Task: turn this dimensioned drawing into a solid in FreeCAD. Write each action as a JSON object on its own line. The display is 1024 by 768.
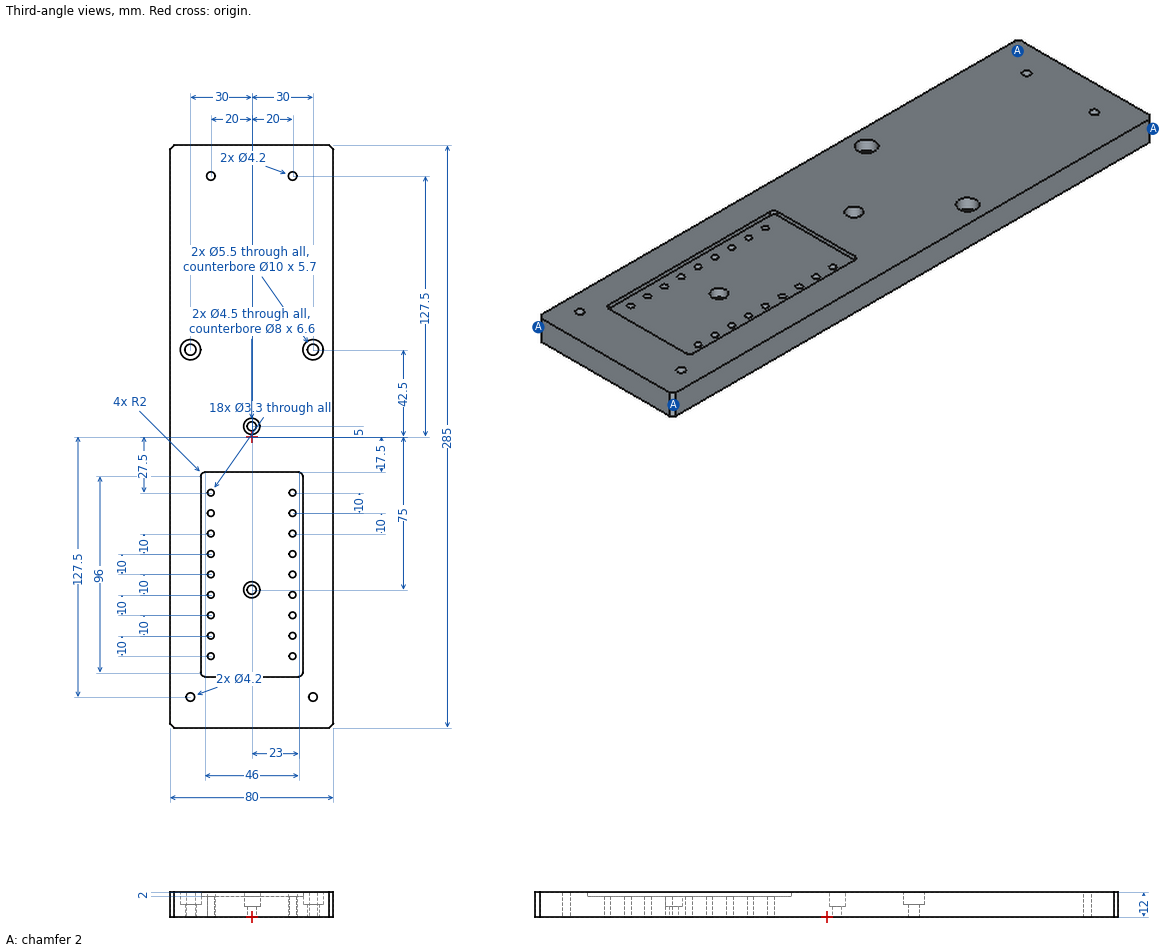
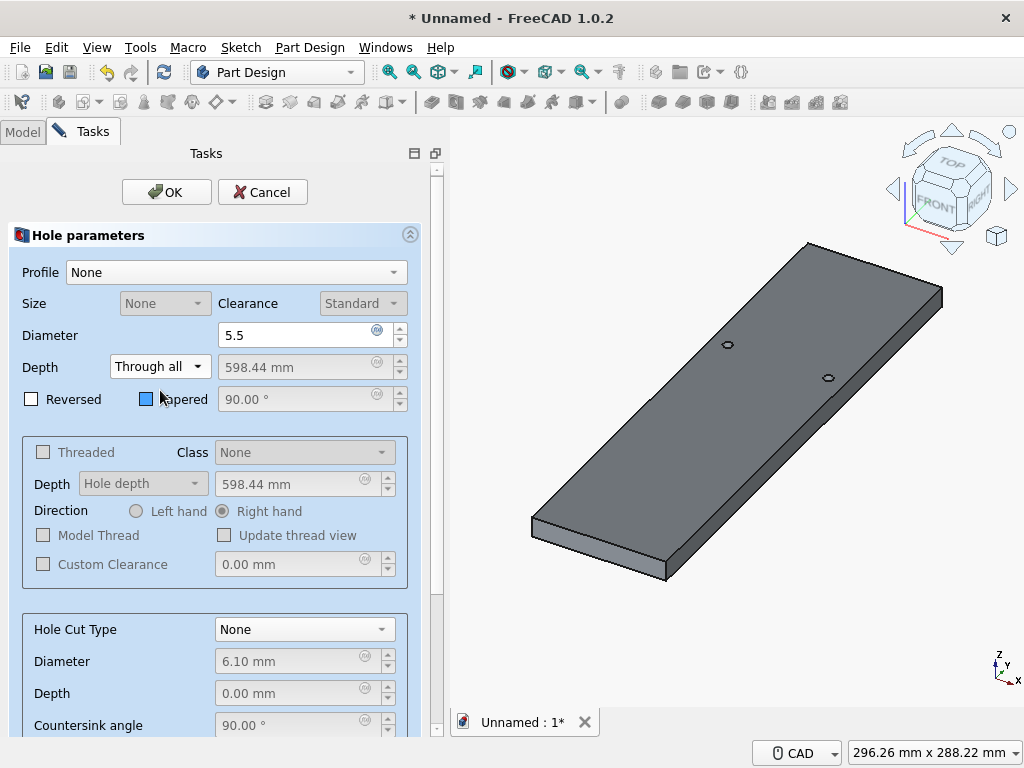
{"action": "left_click", "coordinate": [306, 630]}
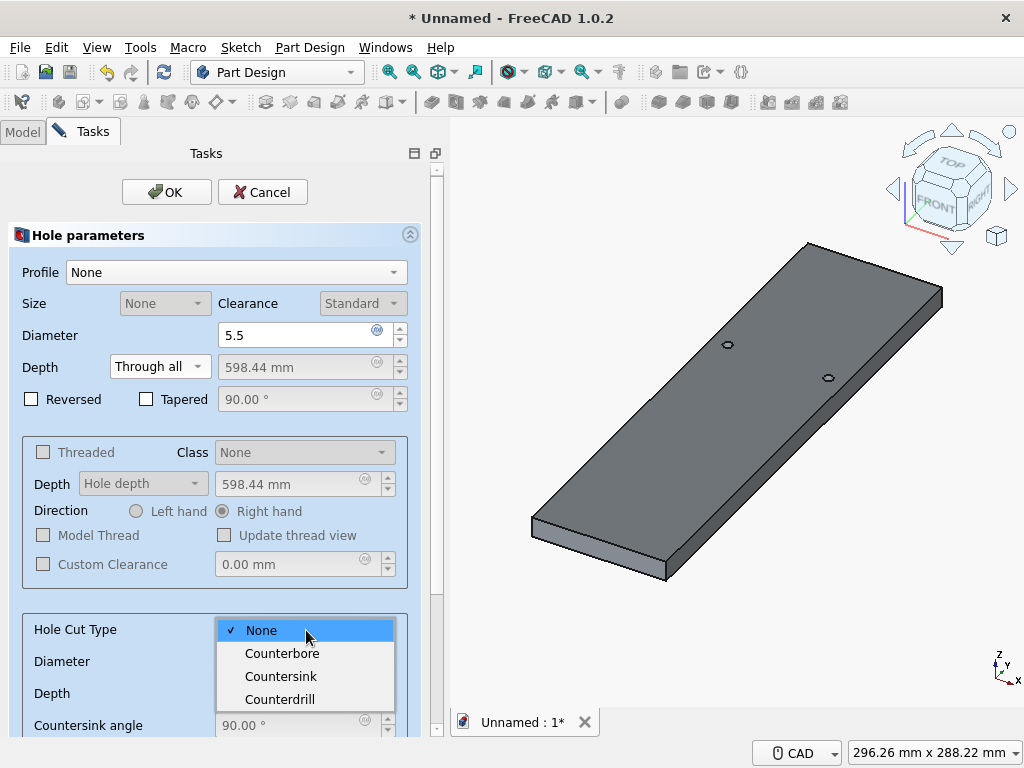
{"action": "left_click", "coordinate": [304, 654]}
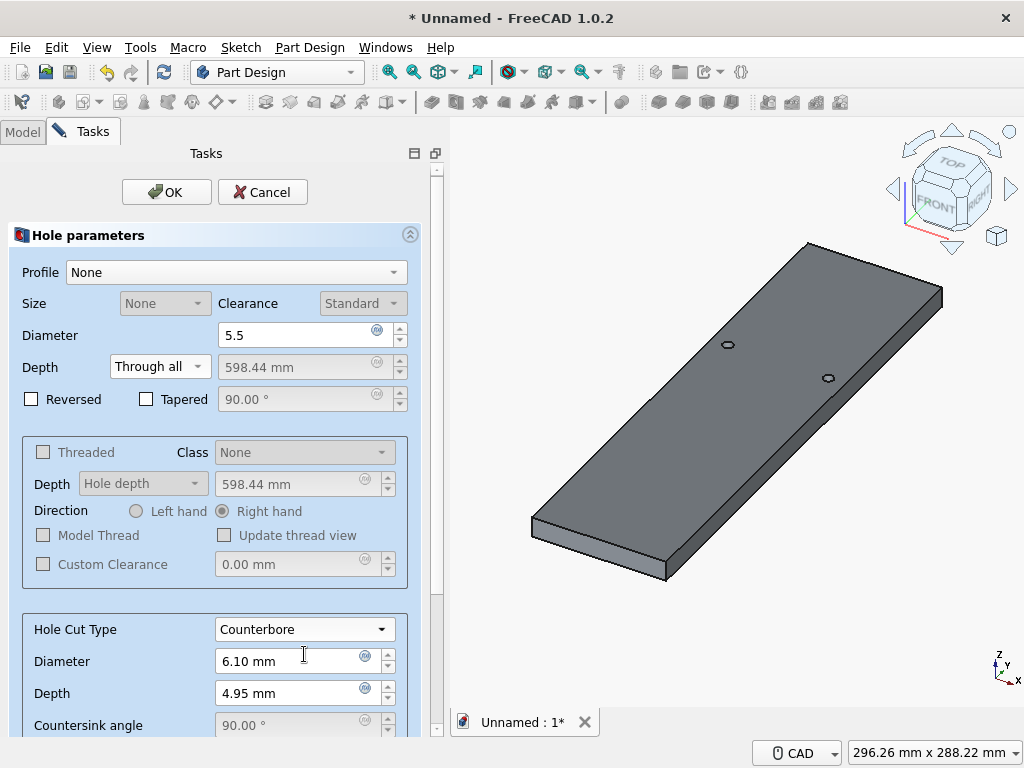
{"action": "triple_click", "coordinate": [298, 661]}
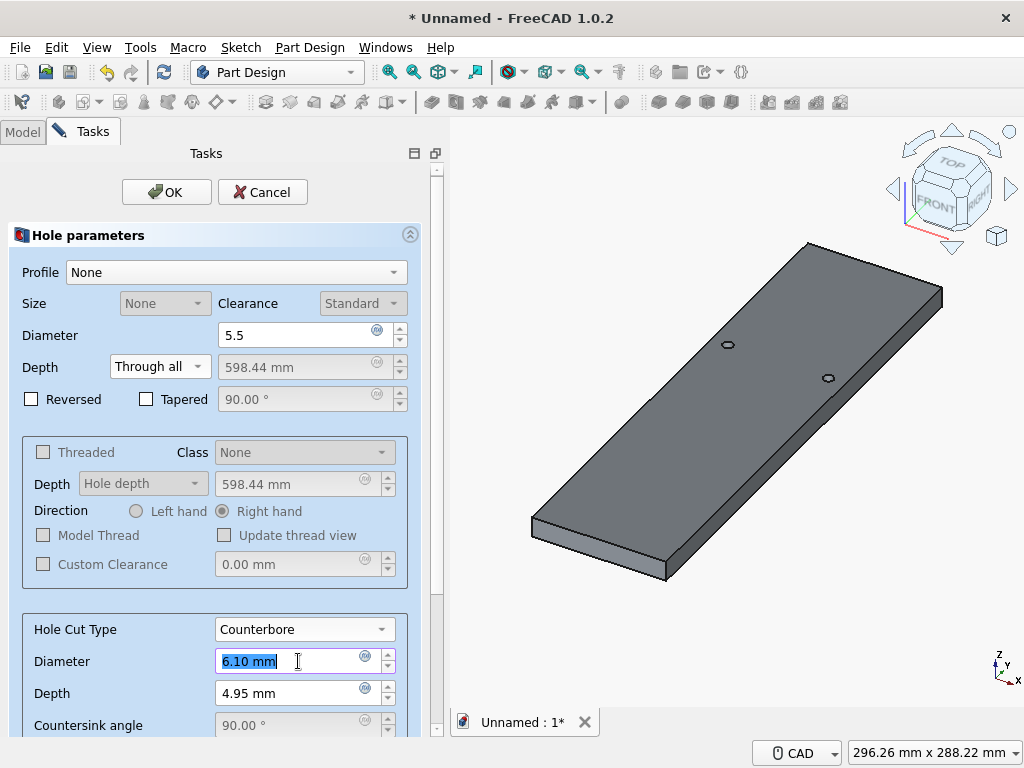
{"action": "type", "text": "10"}
{"action": "key", "text": "Tab"}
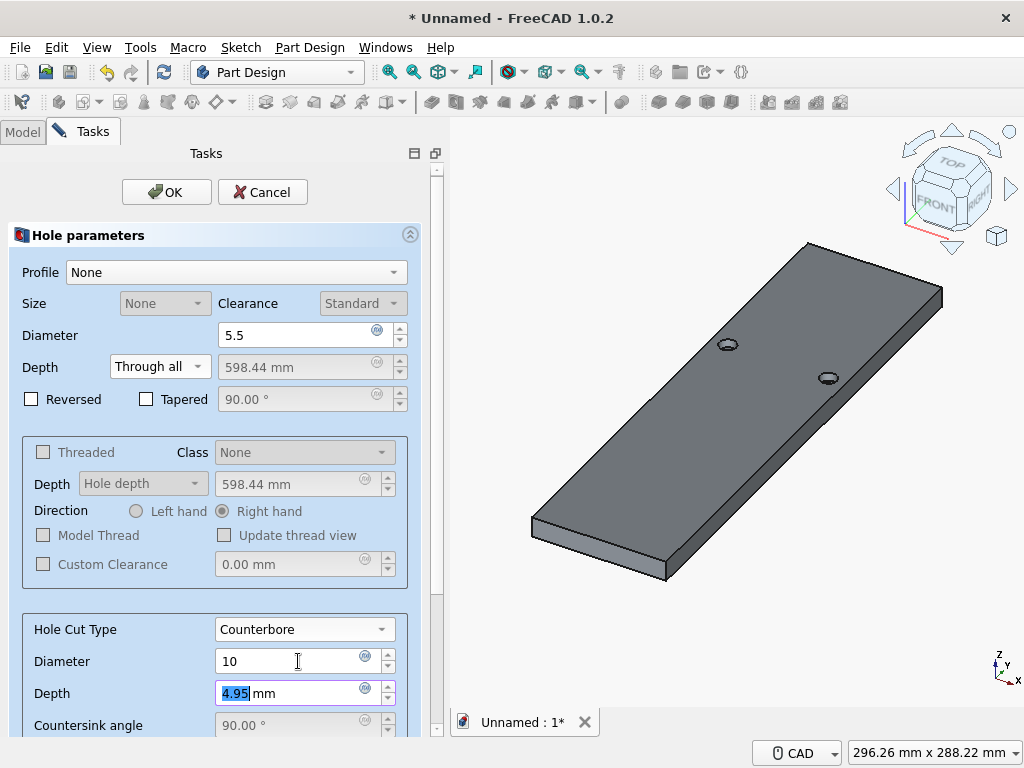
{"action": "type", "text": "5.7"}
{"action": "key", "text": "Tab"}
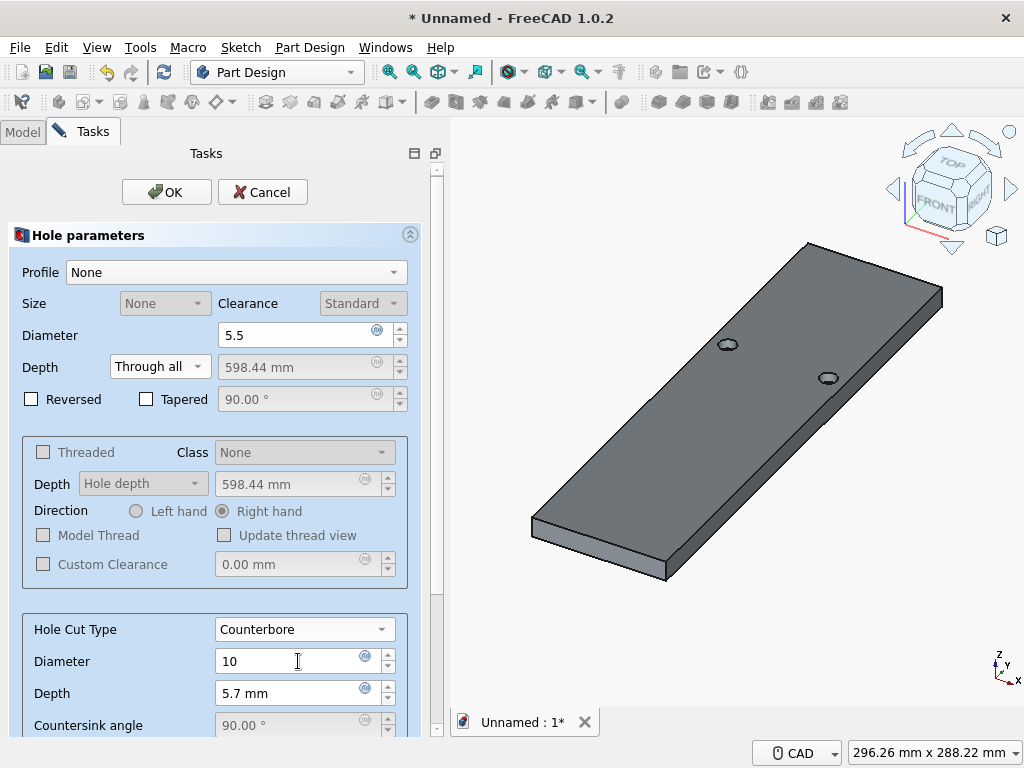
{"action": "left_click", "coordinate": [167, 192]}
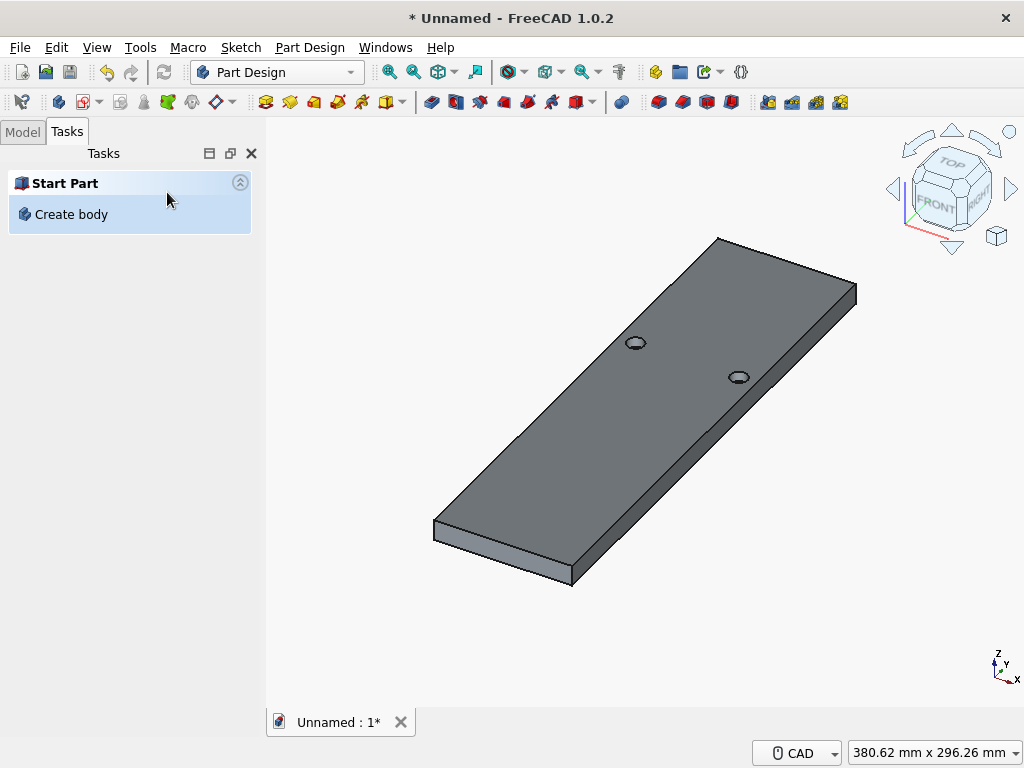
{"action": "key", "text": "5"}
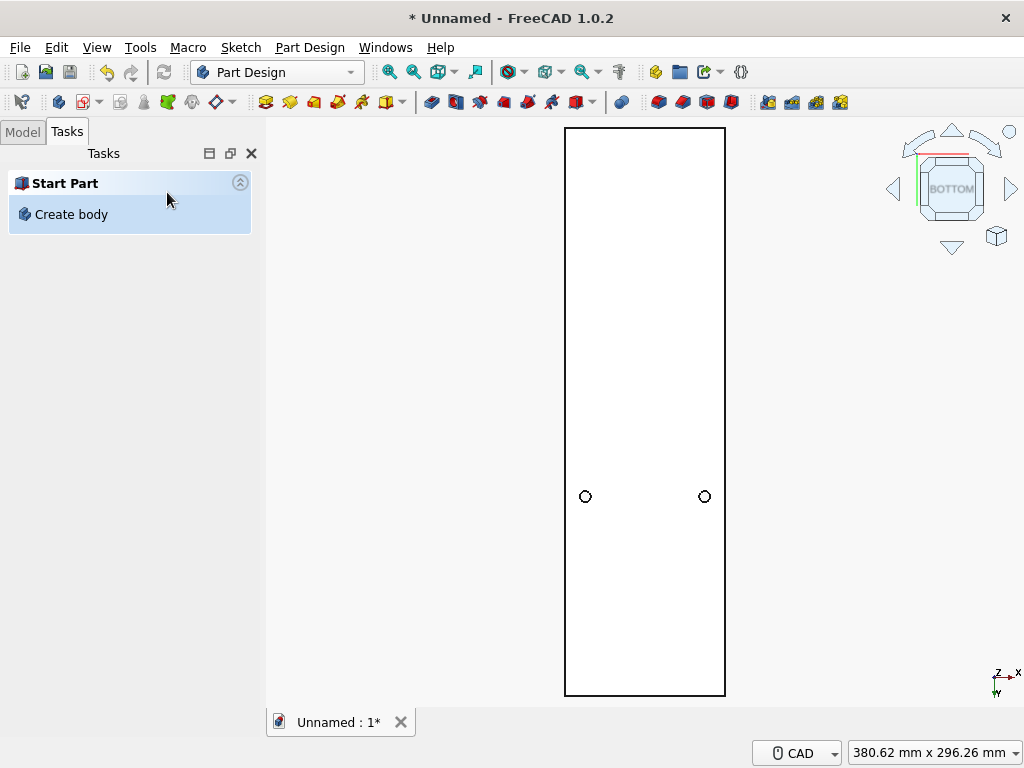
{"action": "left_click", "coordinate": [645, 573]}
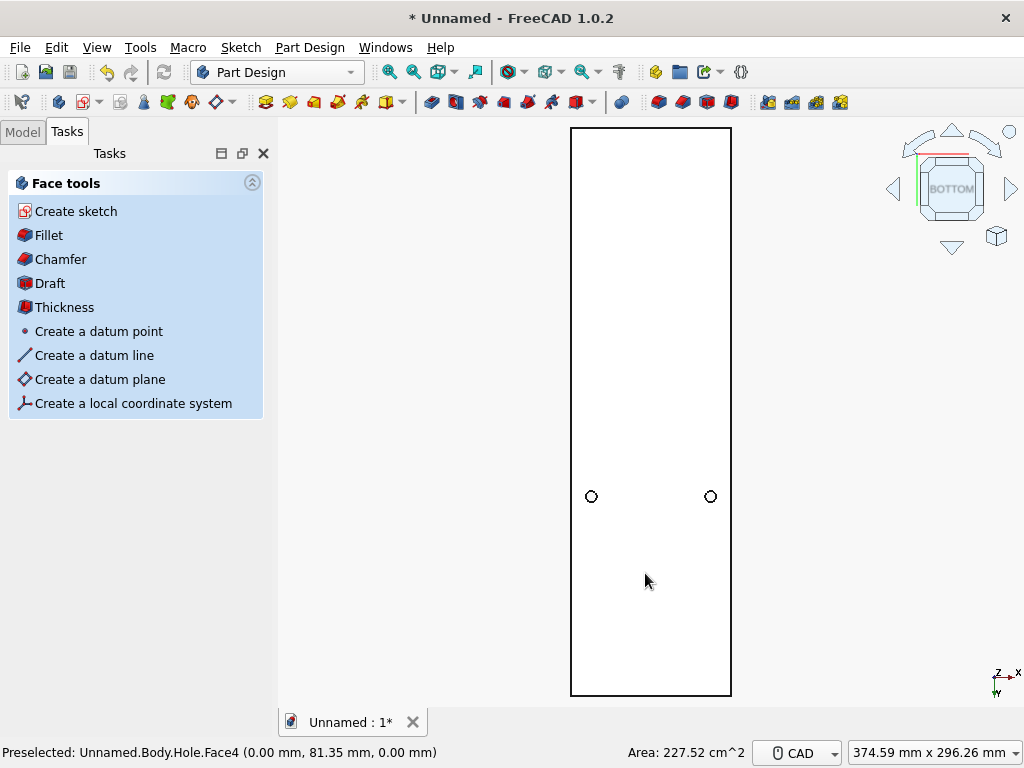
{"action": "left_click", "coordinate": [84, 102]}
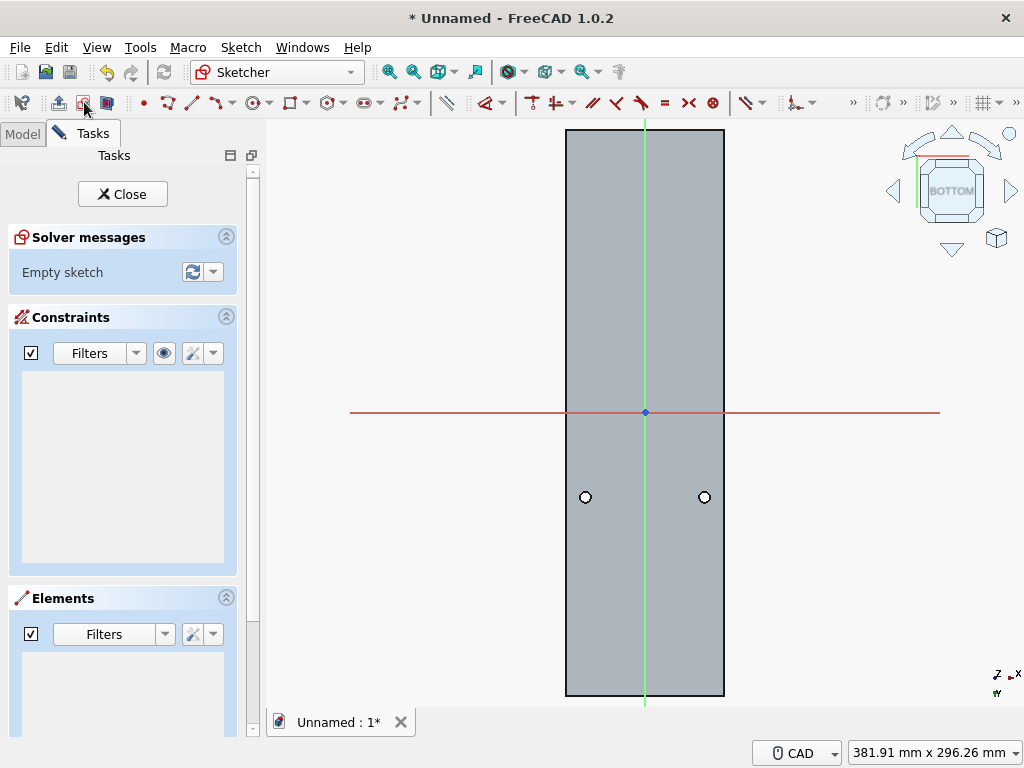
{"action": "scroll", "coordinate": [662, 679], "scroll_direction": "up", "scroll_amount": 8}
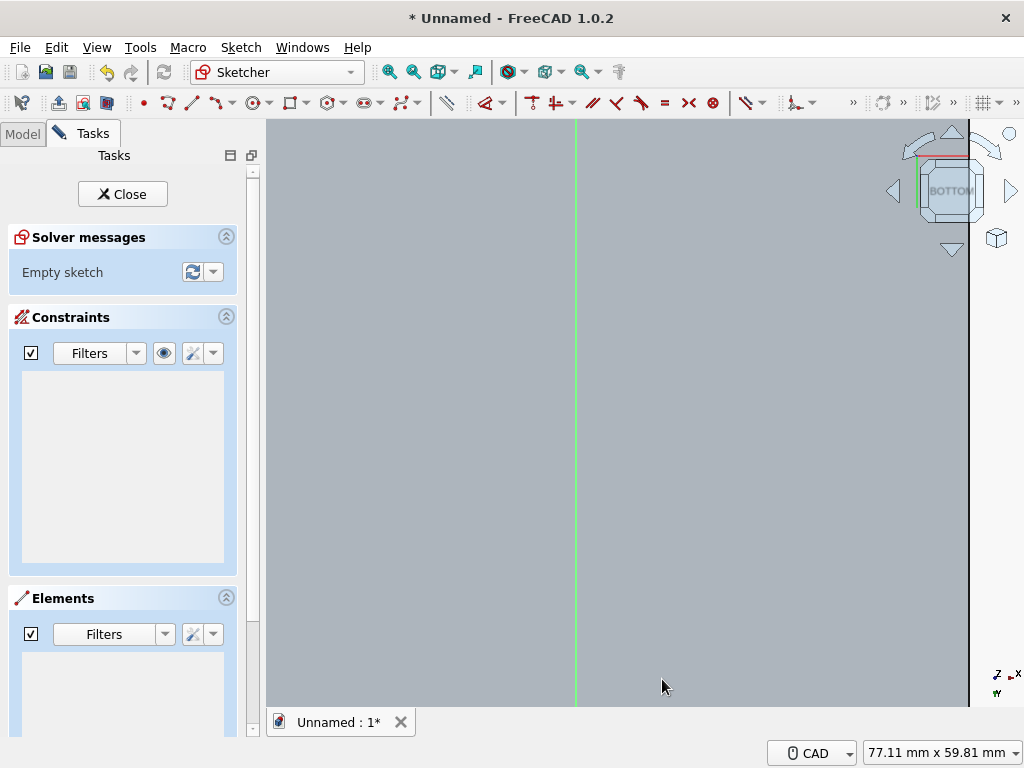
{"action": "key", "text": "g c"}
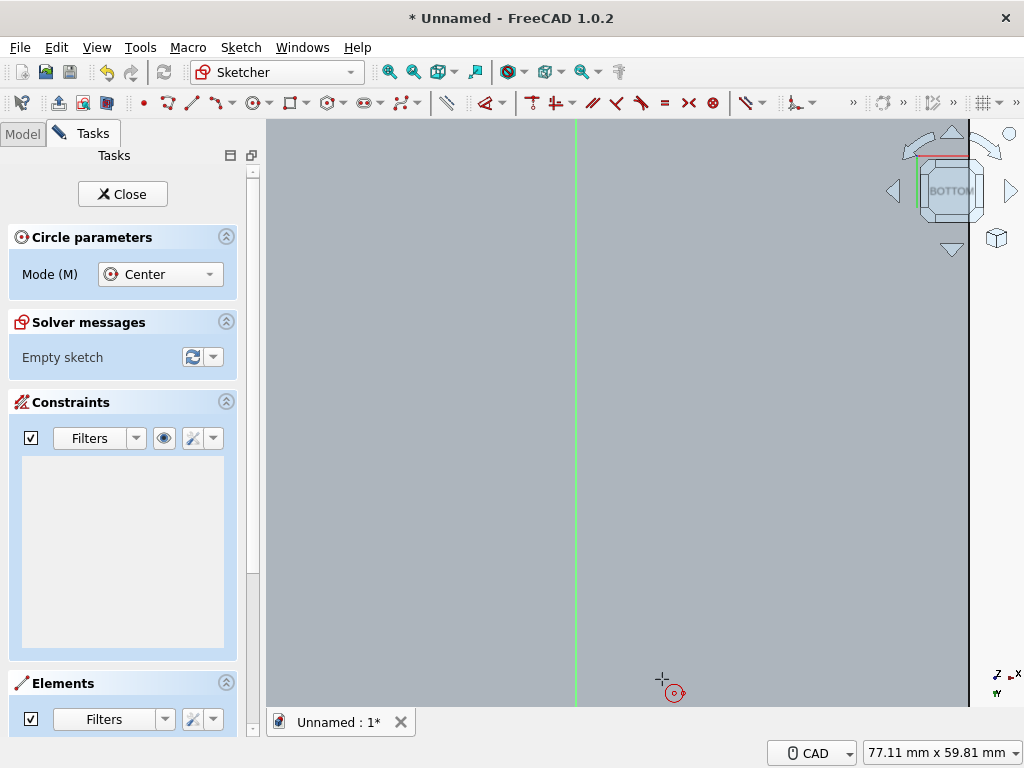
{"action": "left_click", "coordinate": [772, 611]}
{"action": "left_click", "coordinate": [787, 597]}